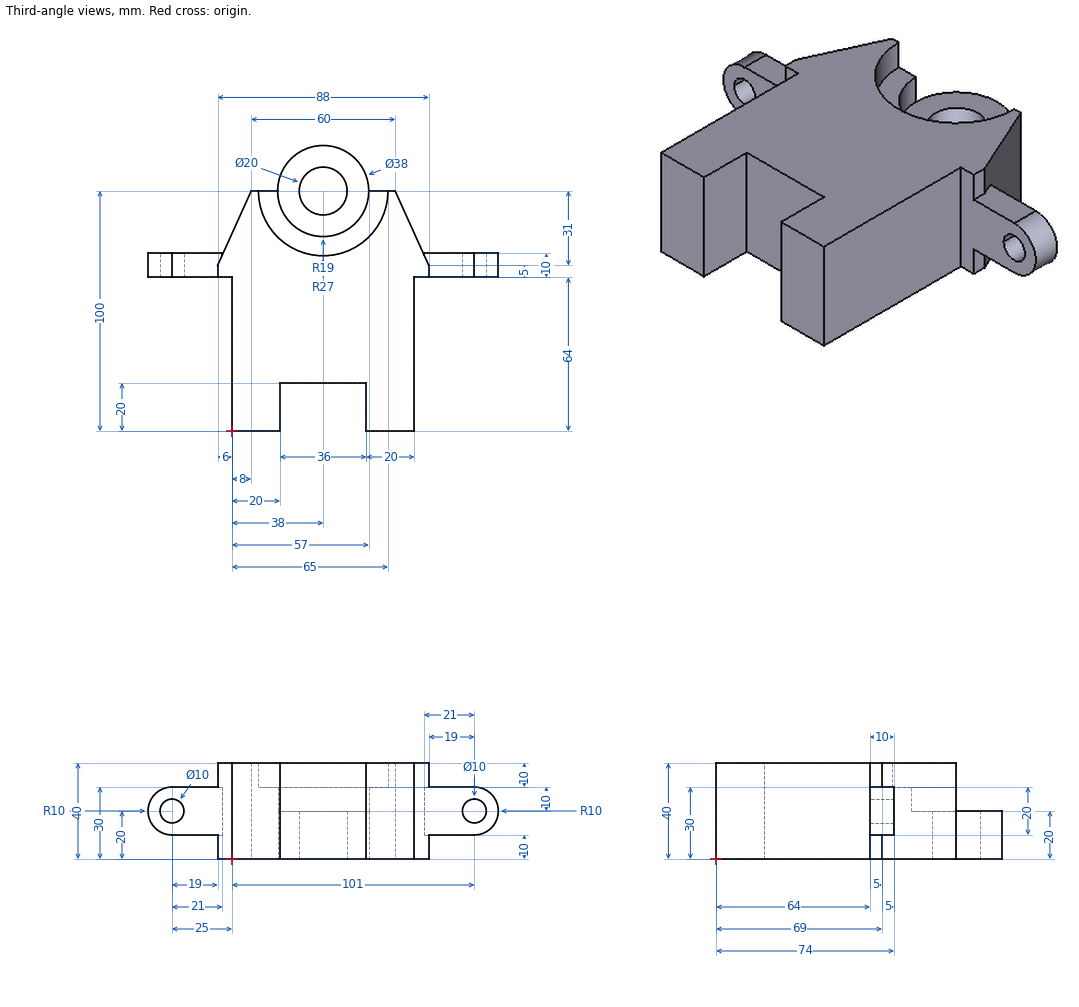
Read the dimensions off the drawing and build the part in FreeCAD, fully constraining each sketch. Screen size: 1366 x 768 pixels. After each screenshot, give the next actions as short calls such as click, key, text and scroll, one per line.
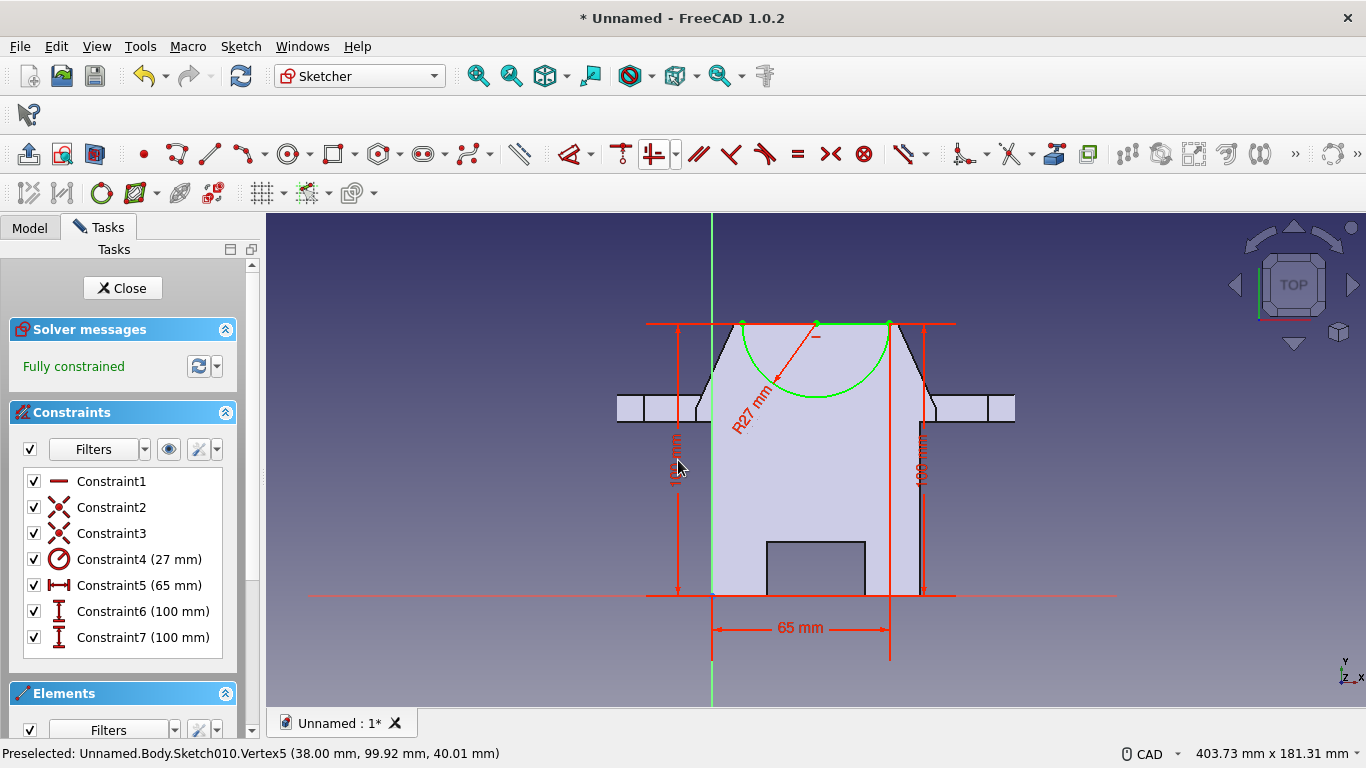
click(123, 288)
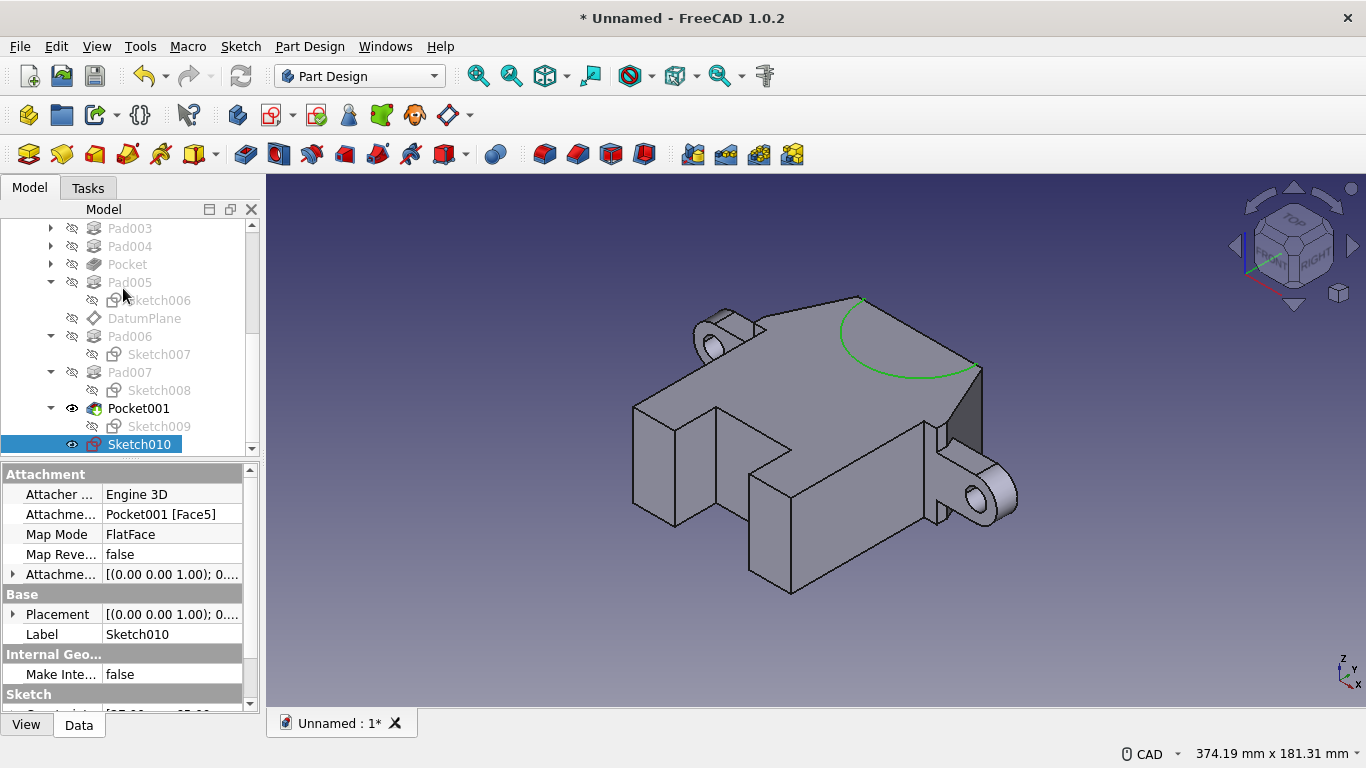
click(246, 154)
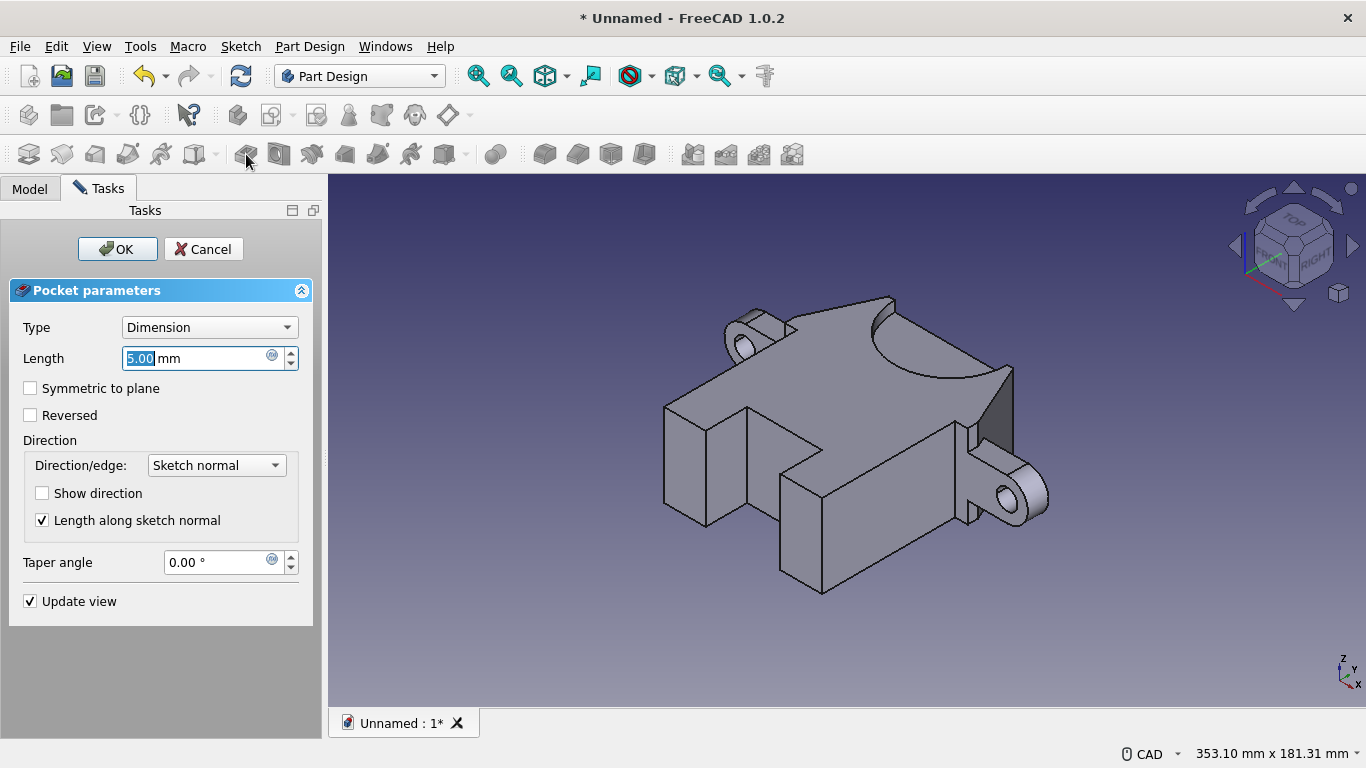
text(10)
key(Tab)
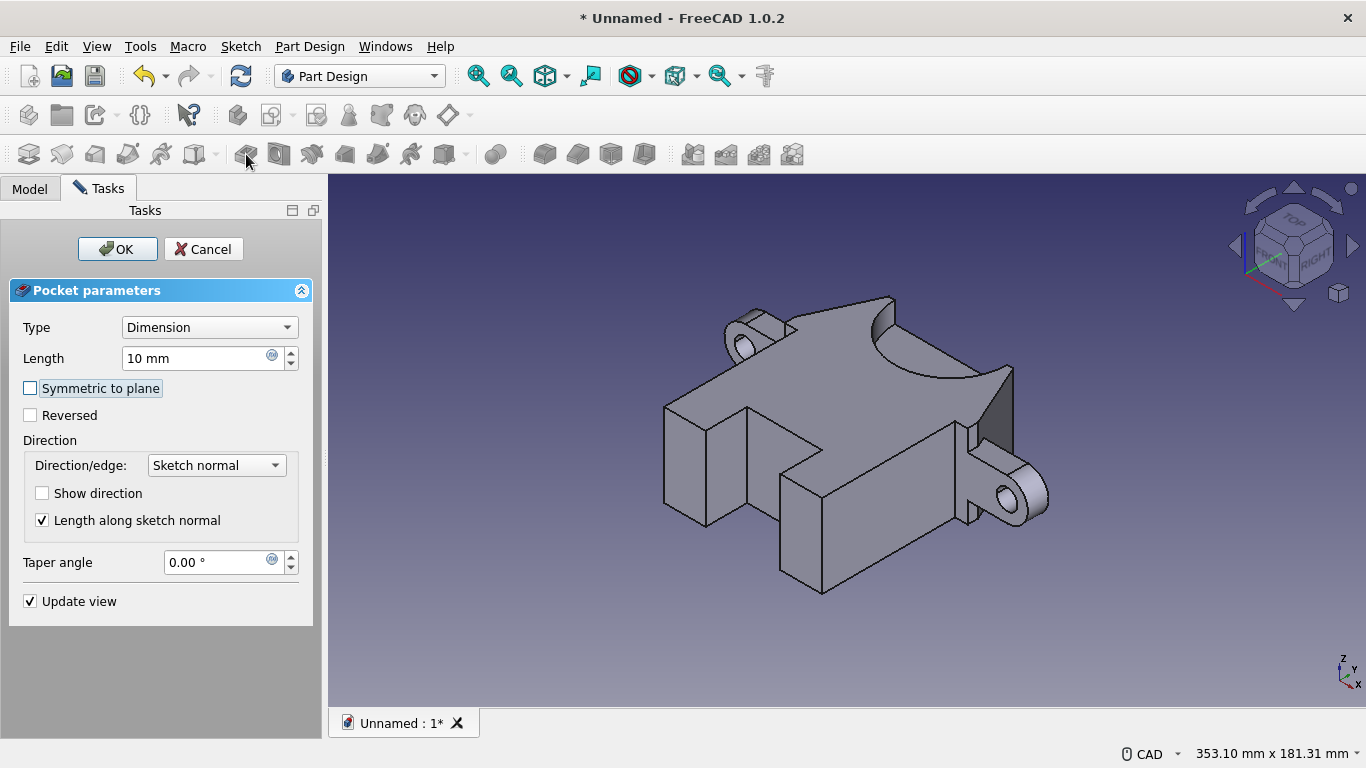
click(118, 249)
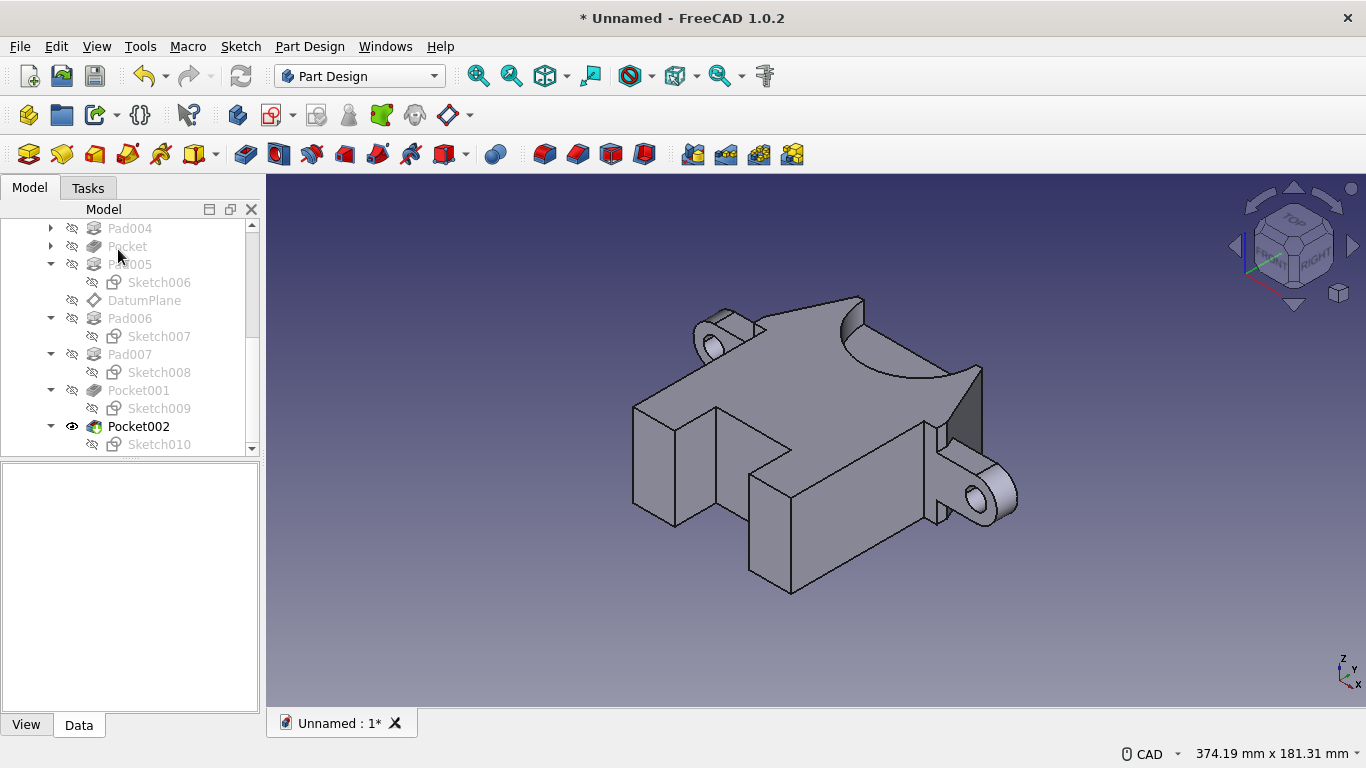
click(900, 367)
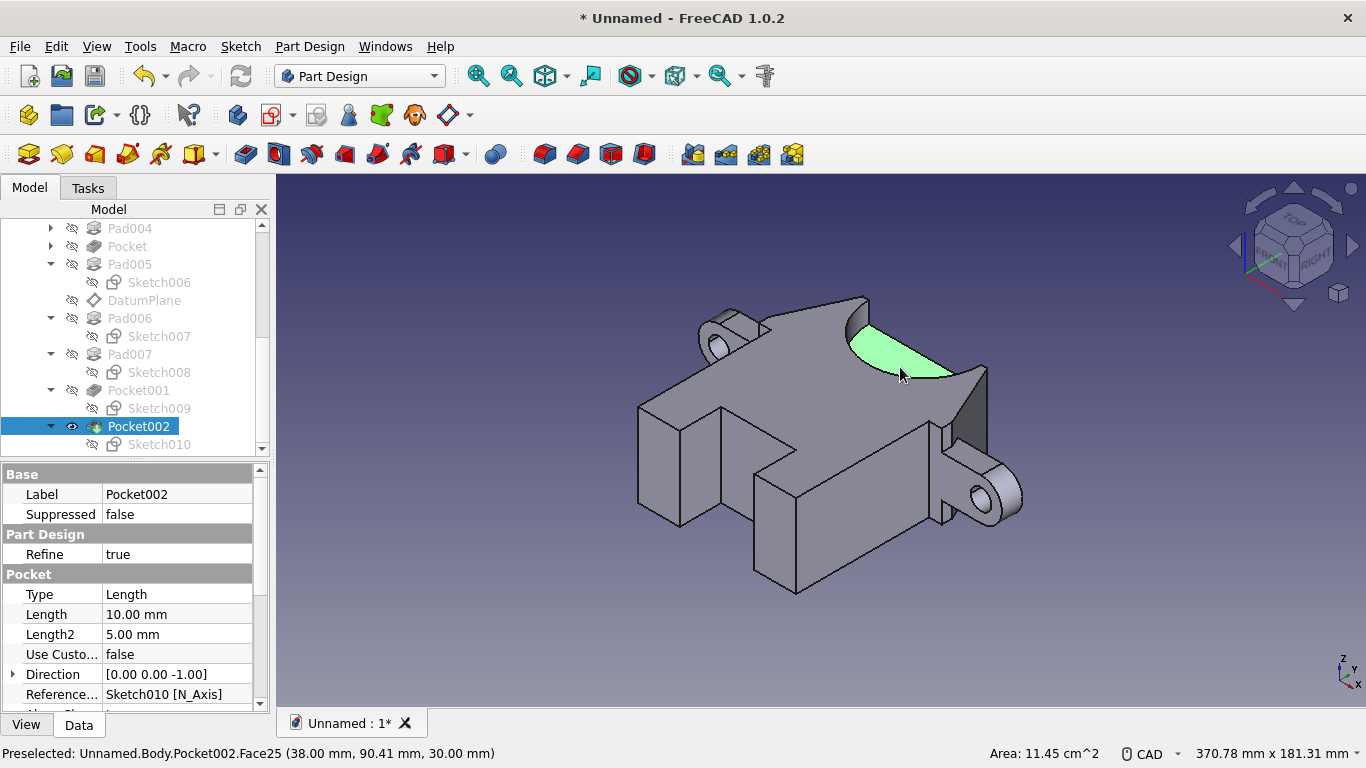
click(270, 116)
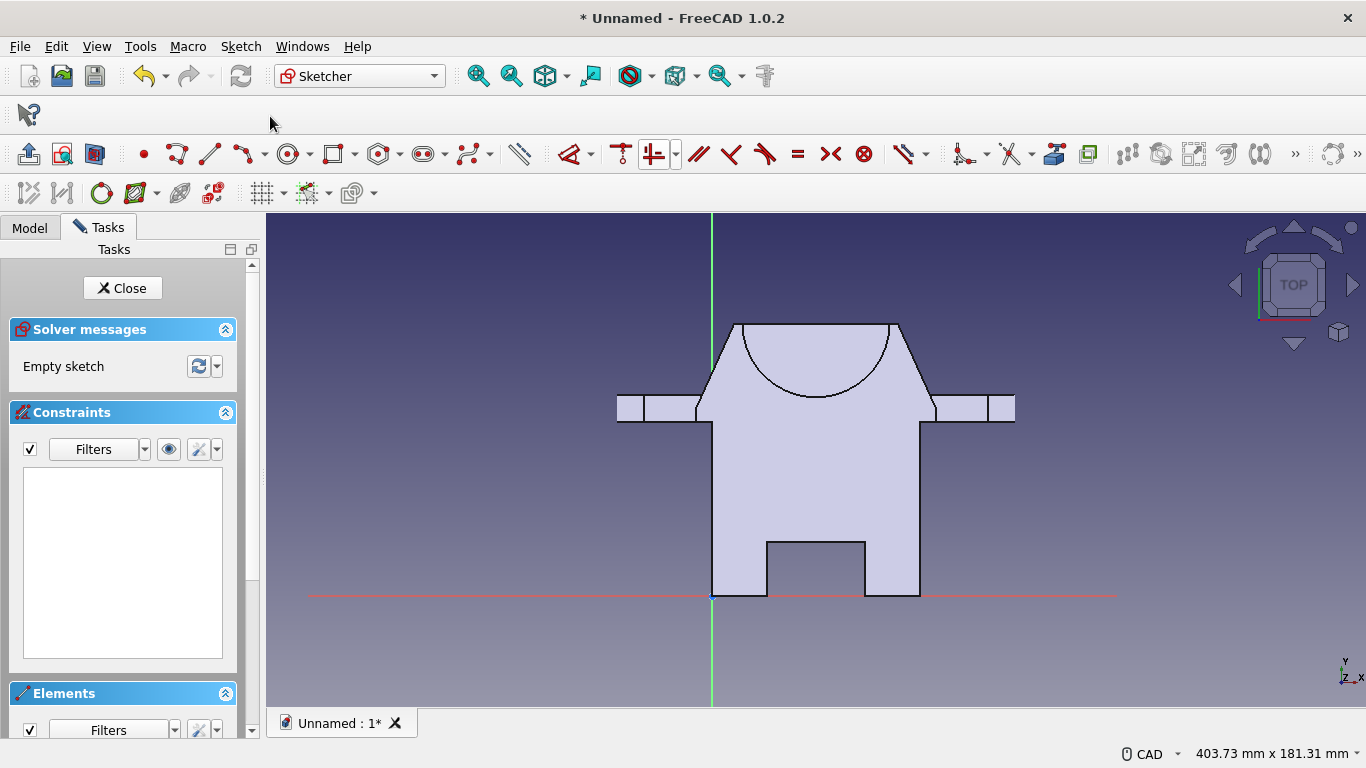
click(95, 154)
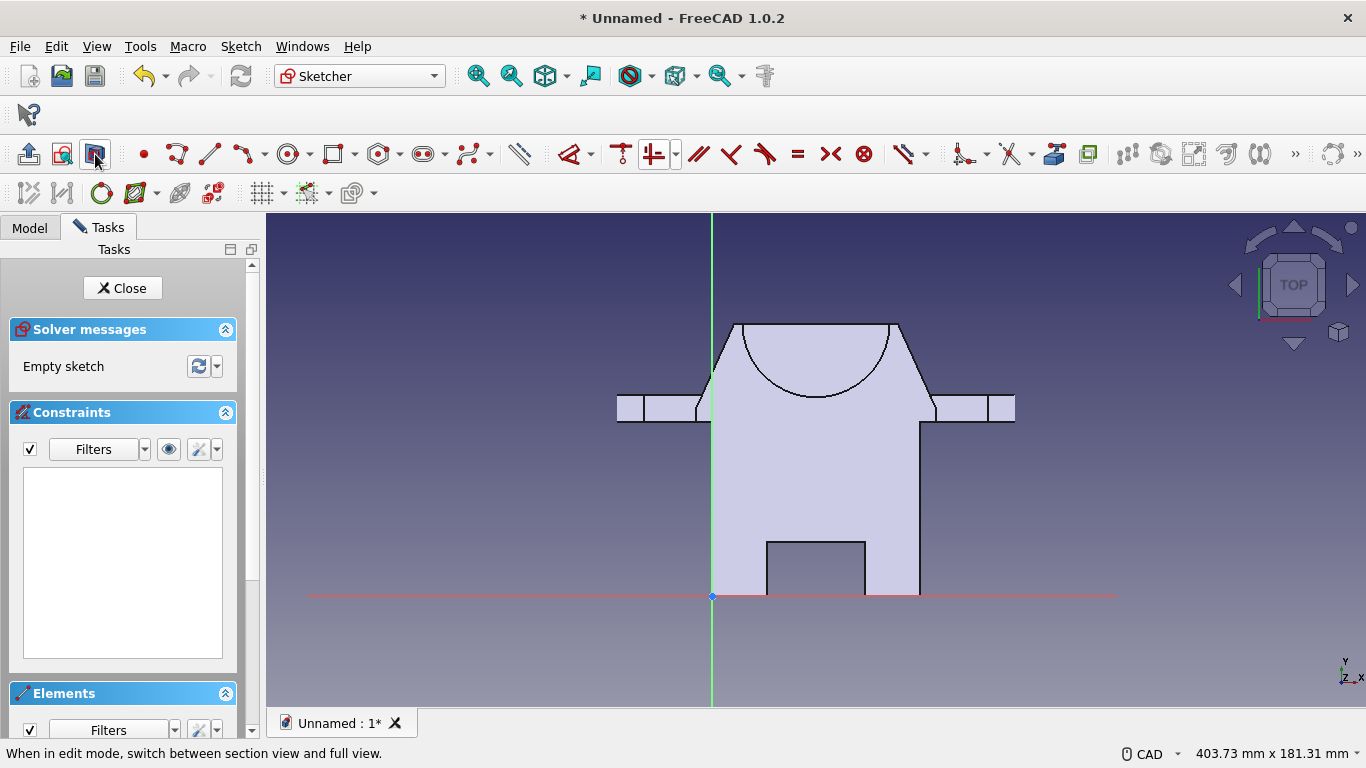
scroll(830, 328, up, 9)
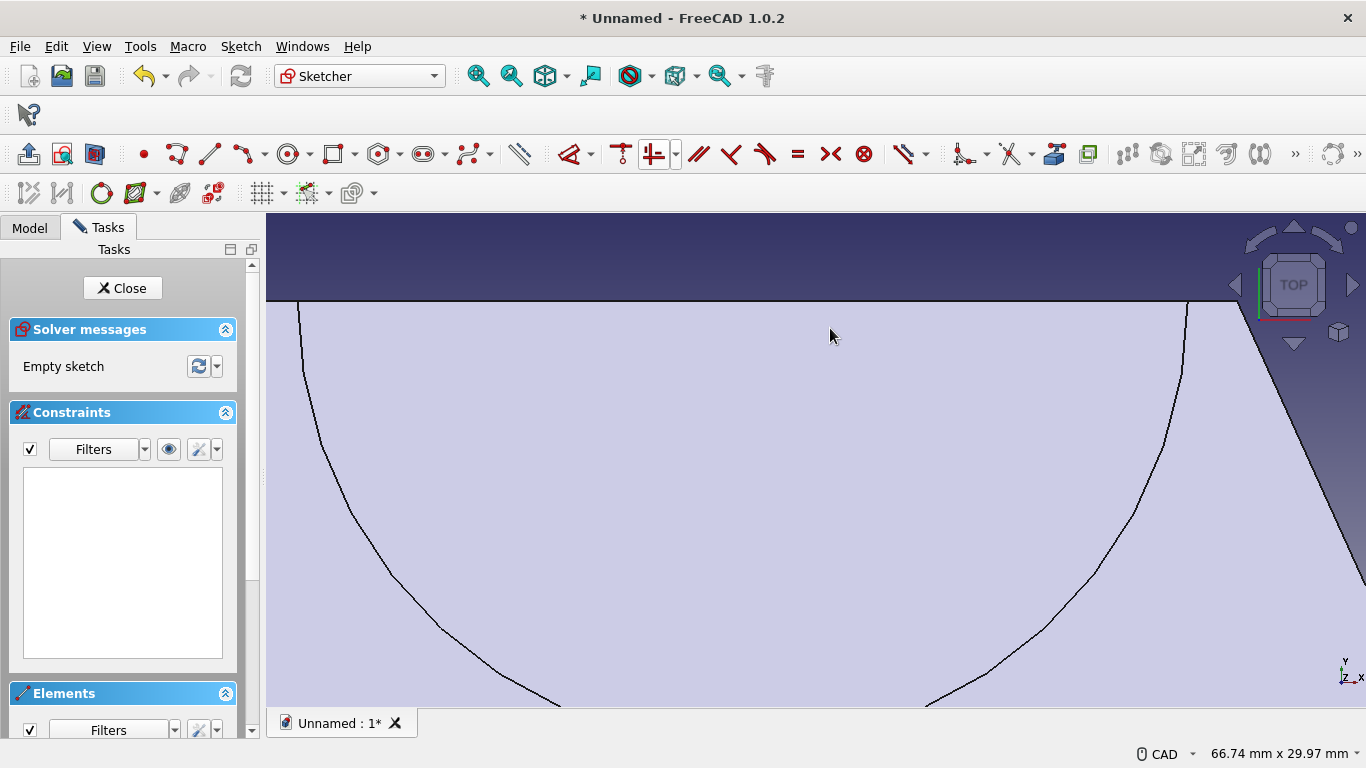
click(210, 154)